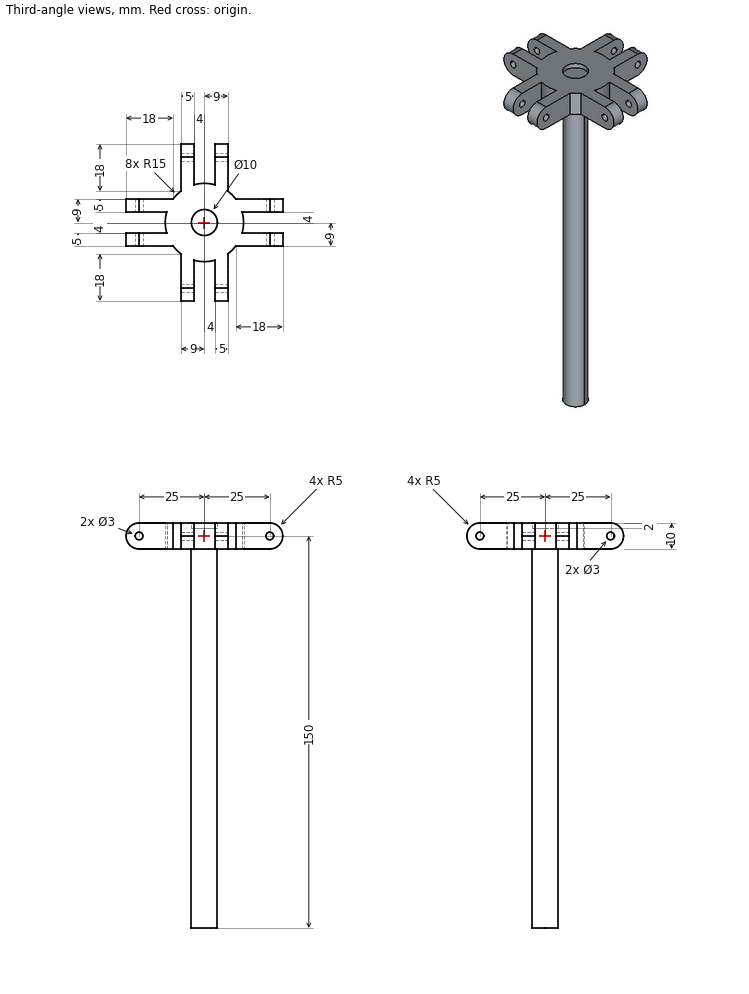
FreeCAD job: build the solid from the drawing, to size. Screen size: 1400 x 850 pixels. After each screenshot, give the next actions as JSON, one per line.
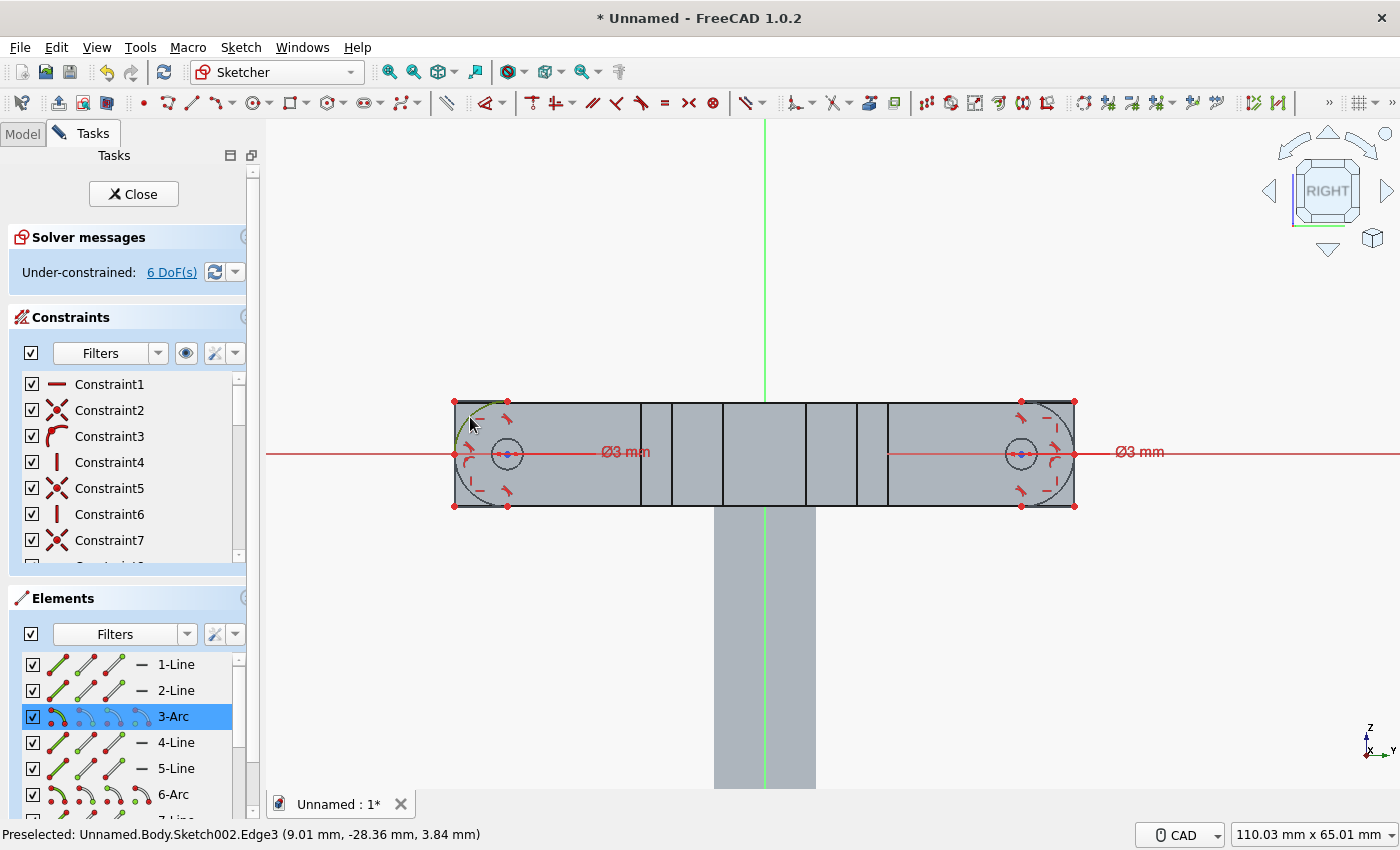
{"action": "left_click", "coordinate": [470, 491]}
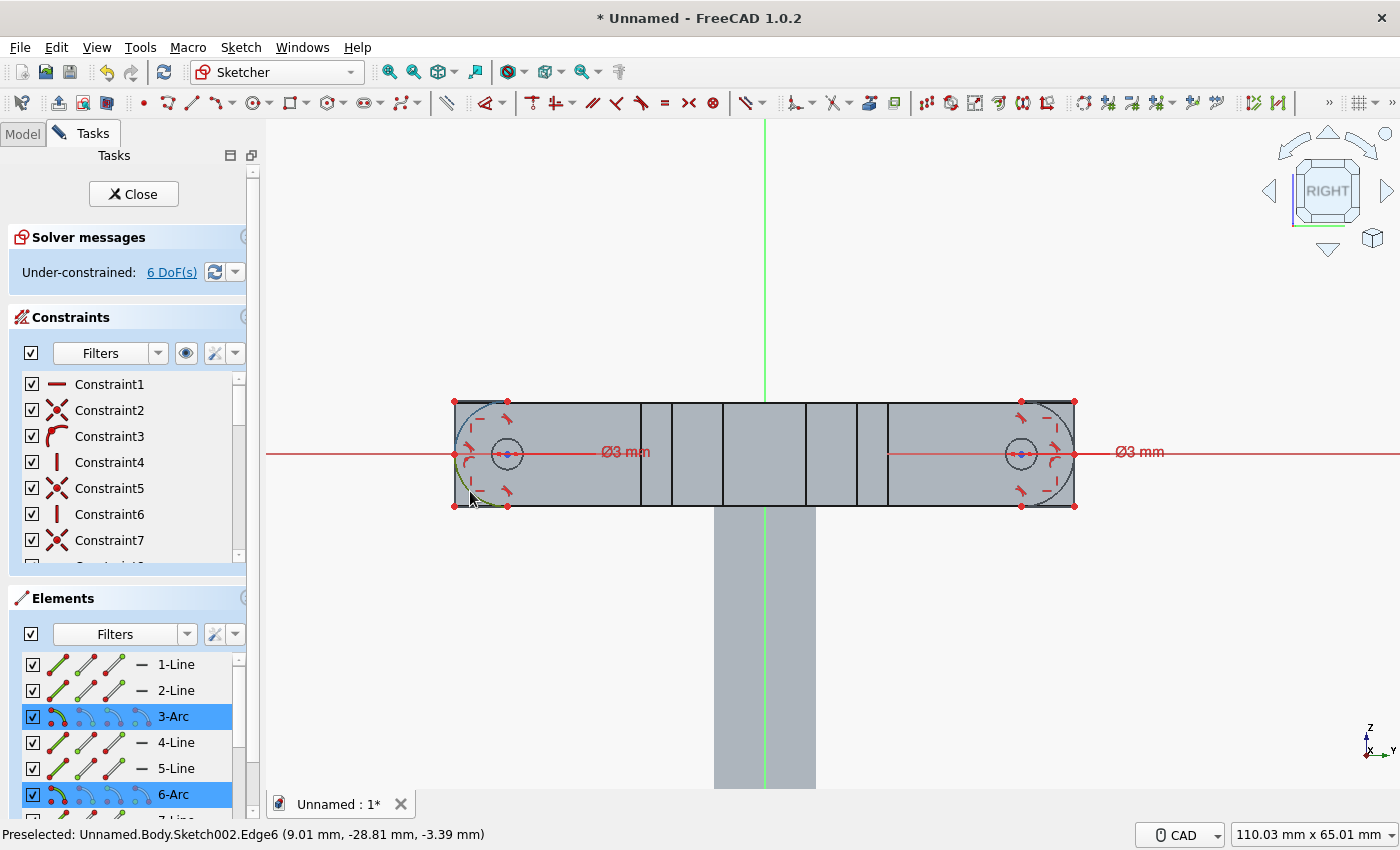
{"action": "left_click", "coordinate": [1059, 417]}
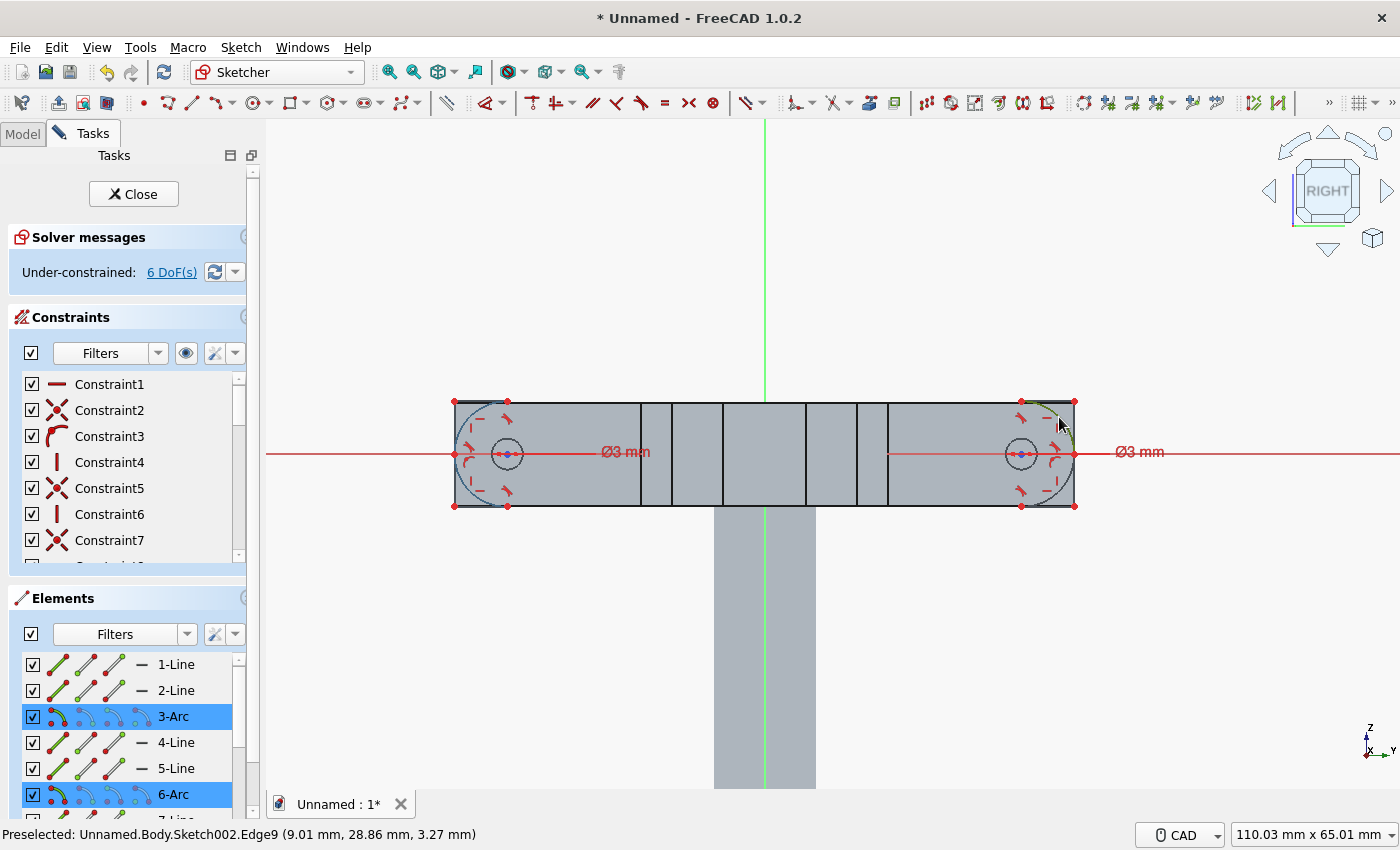
{"action": "left_click", "coordinate": [1059, 491]}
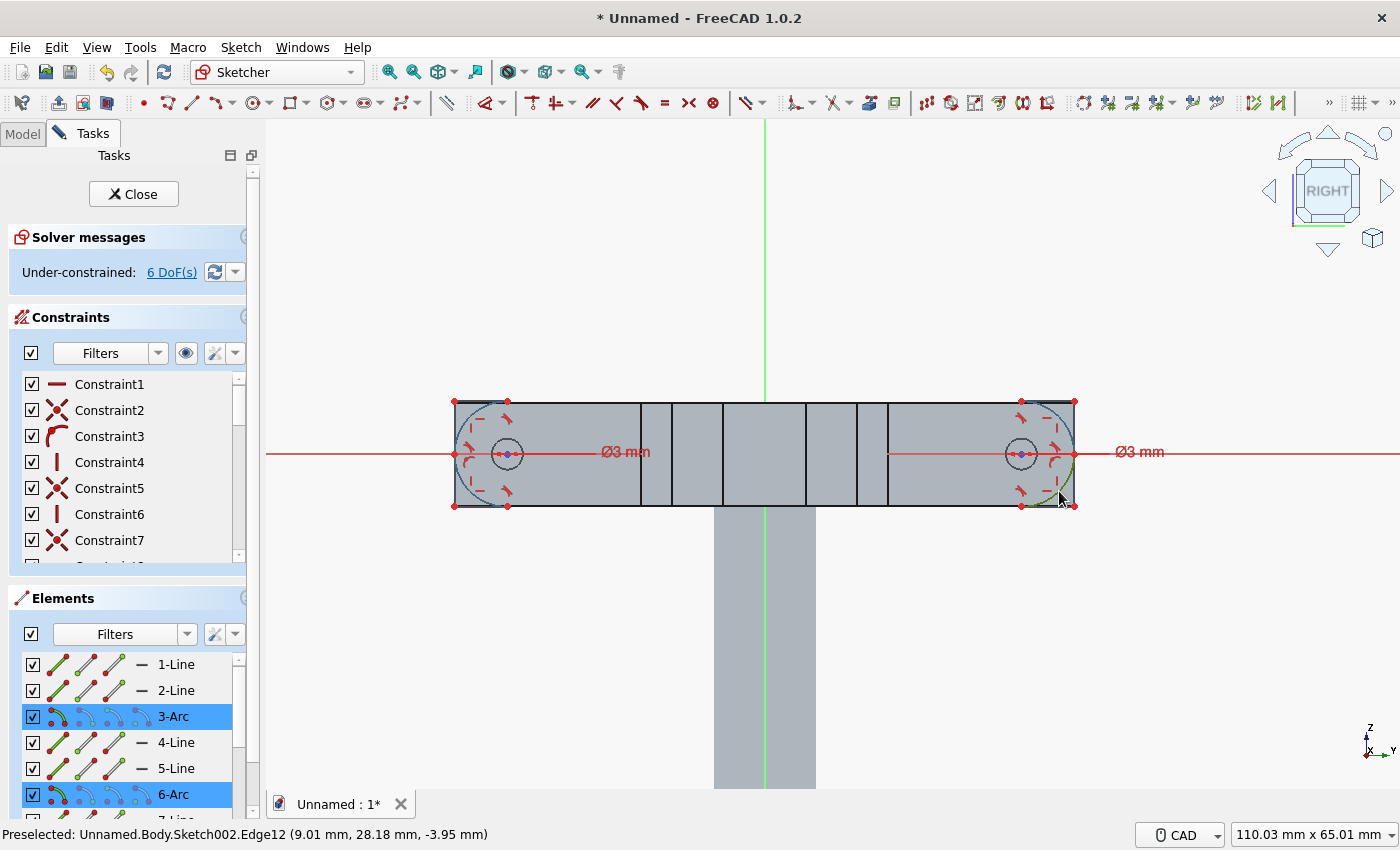
{"action": "key", "text": "e"}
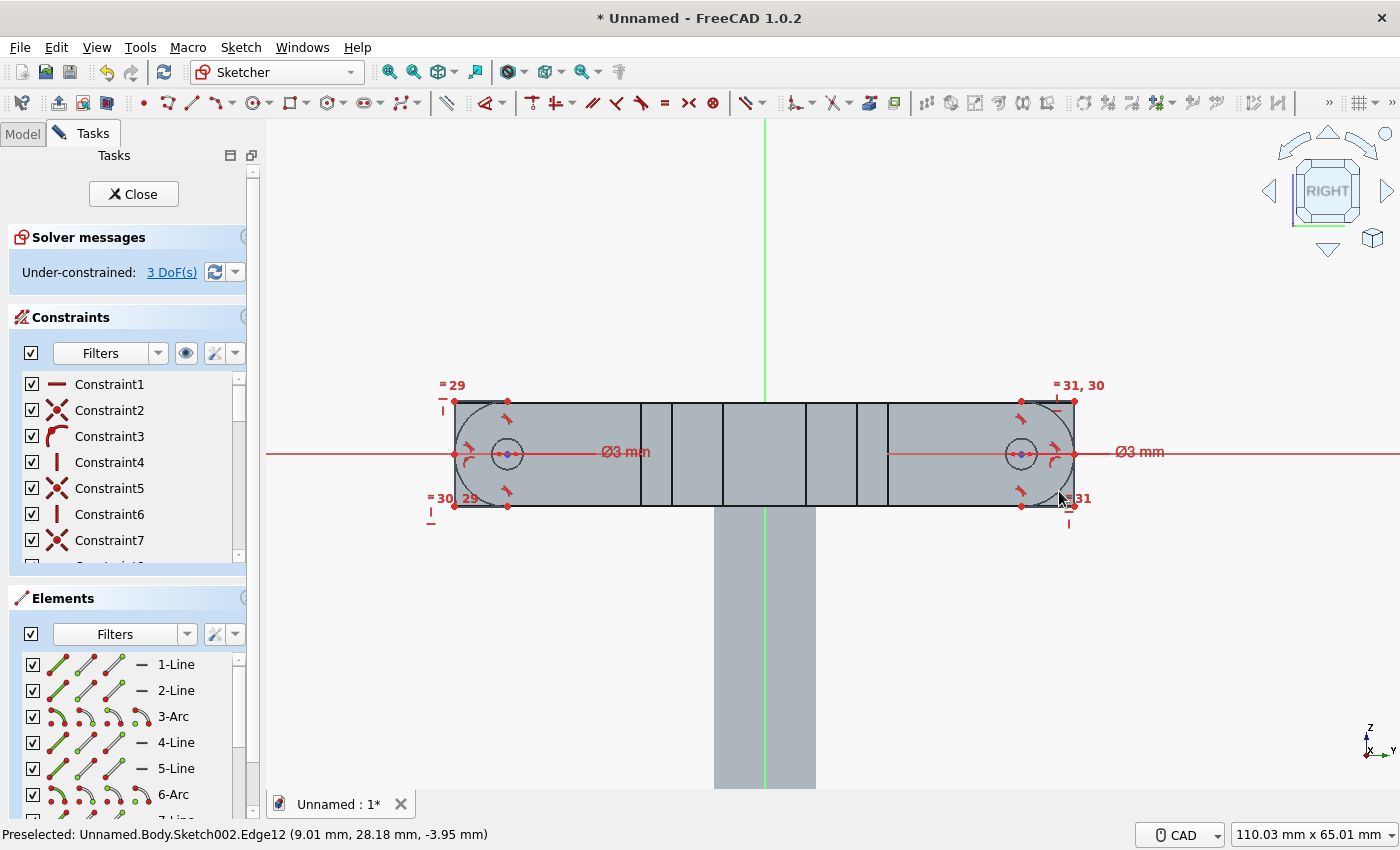
{"action": "key", "text": "d"}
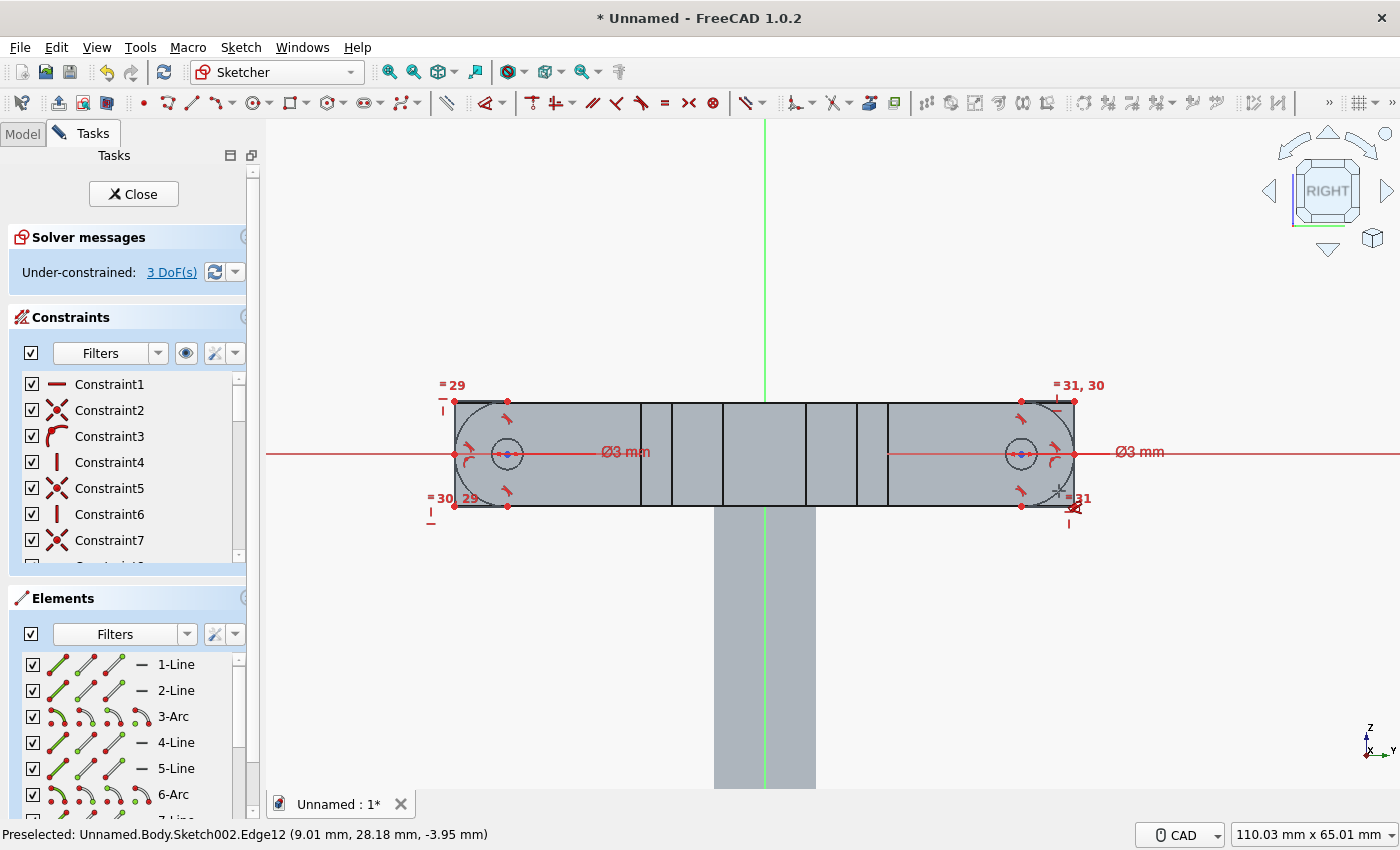
{"action": "left_click", "coordinate": [470, 417]}
{"action": "left_click", "coordinate": [483, 373]}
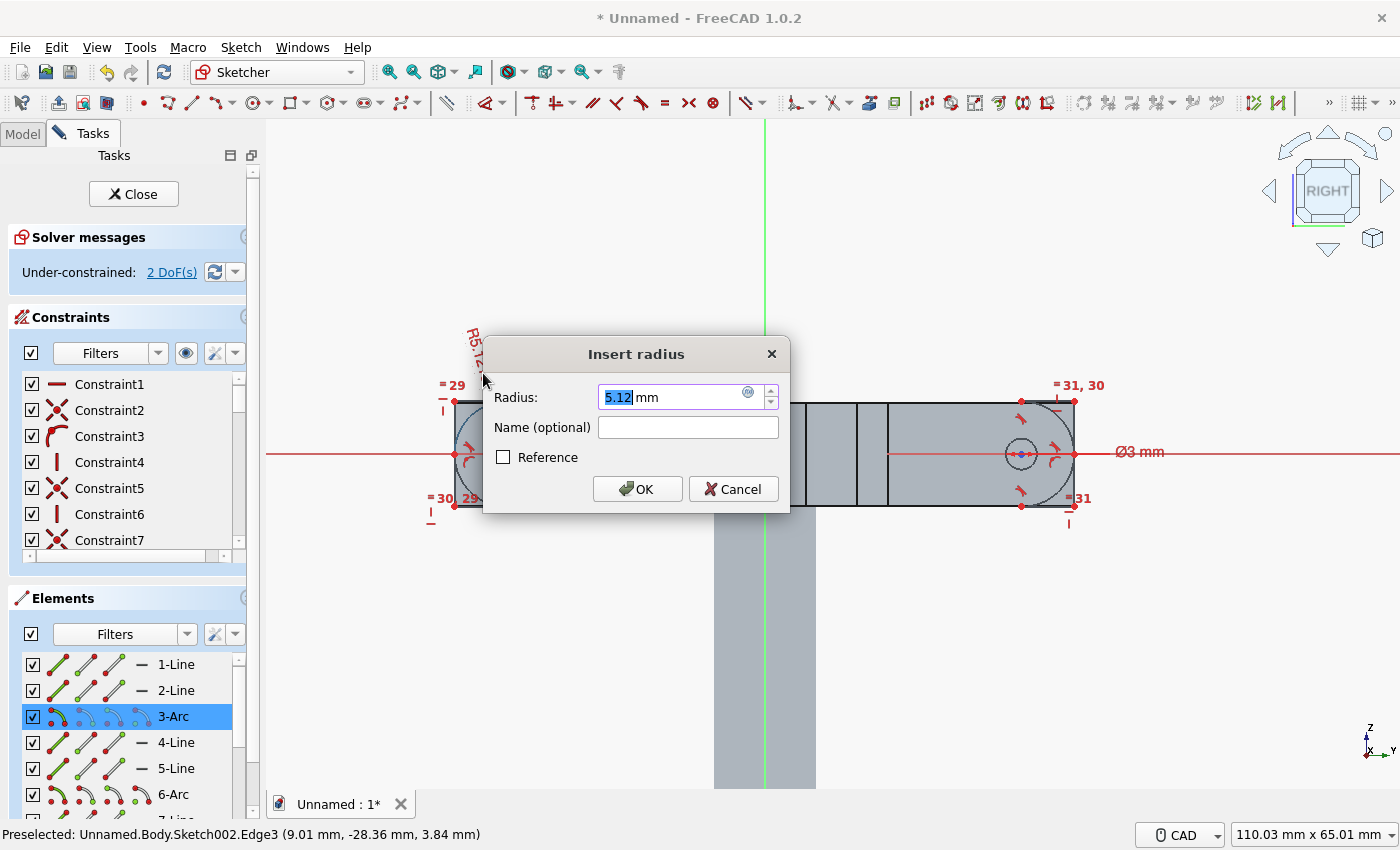
{"action": "type", "text": "5"}
{"action": "key", "text": "Return"}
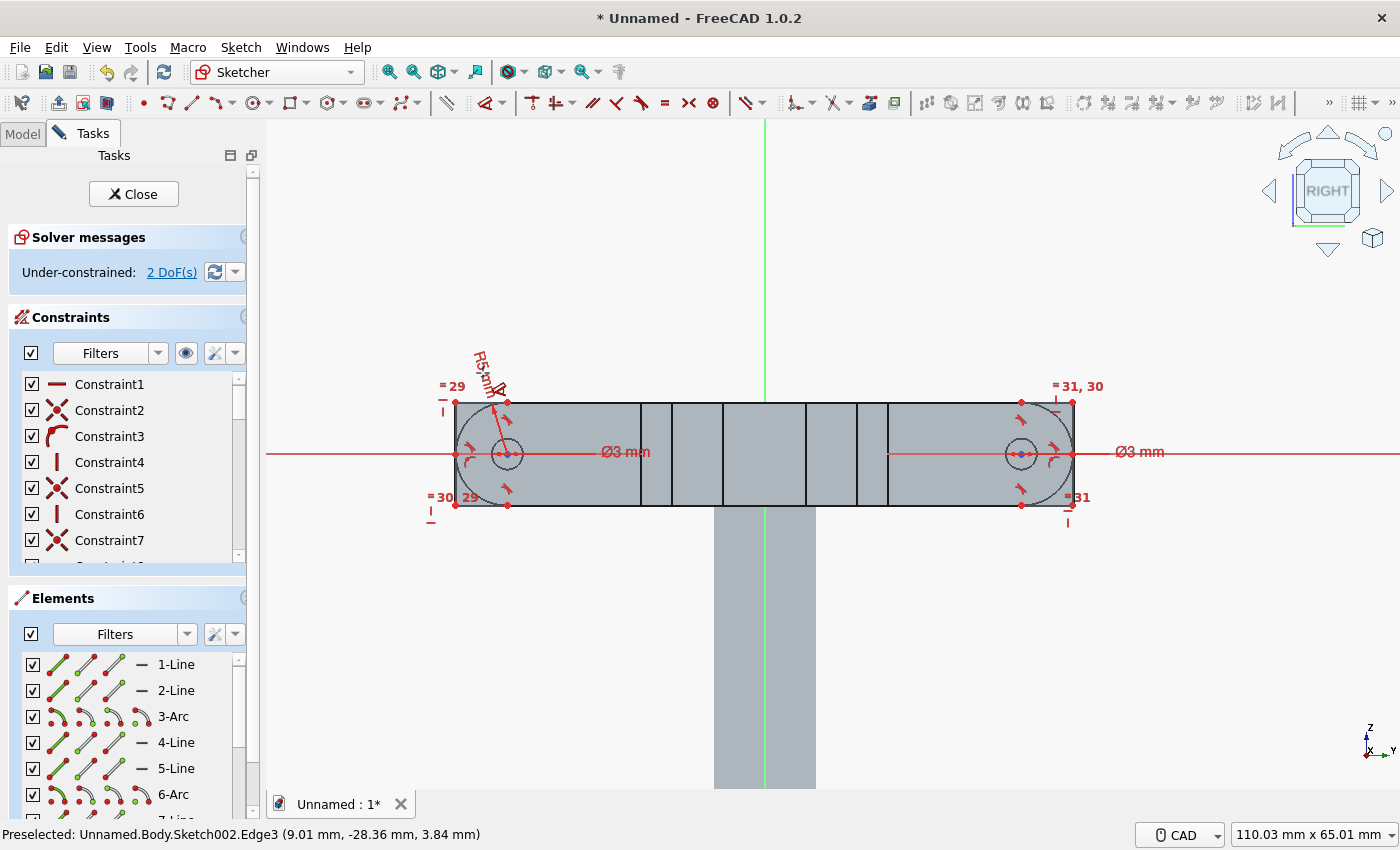
{"action": "left_click", "coordinate": [1021, 454]}
{"action": "left_click", "coordinate": [893, 488]}